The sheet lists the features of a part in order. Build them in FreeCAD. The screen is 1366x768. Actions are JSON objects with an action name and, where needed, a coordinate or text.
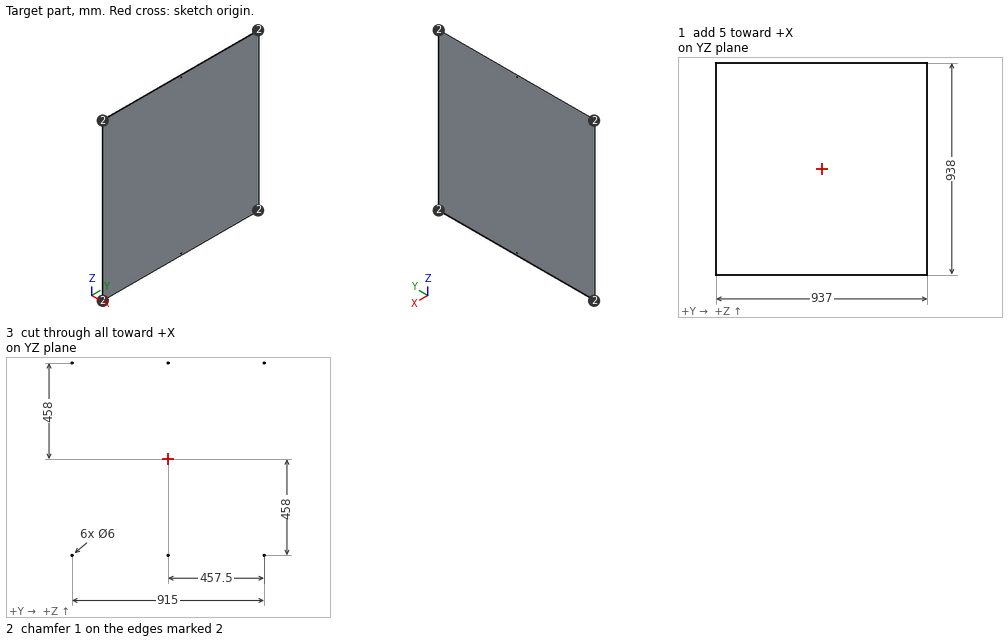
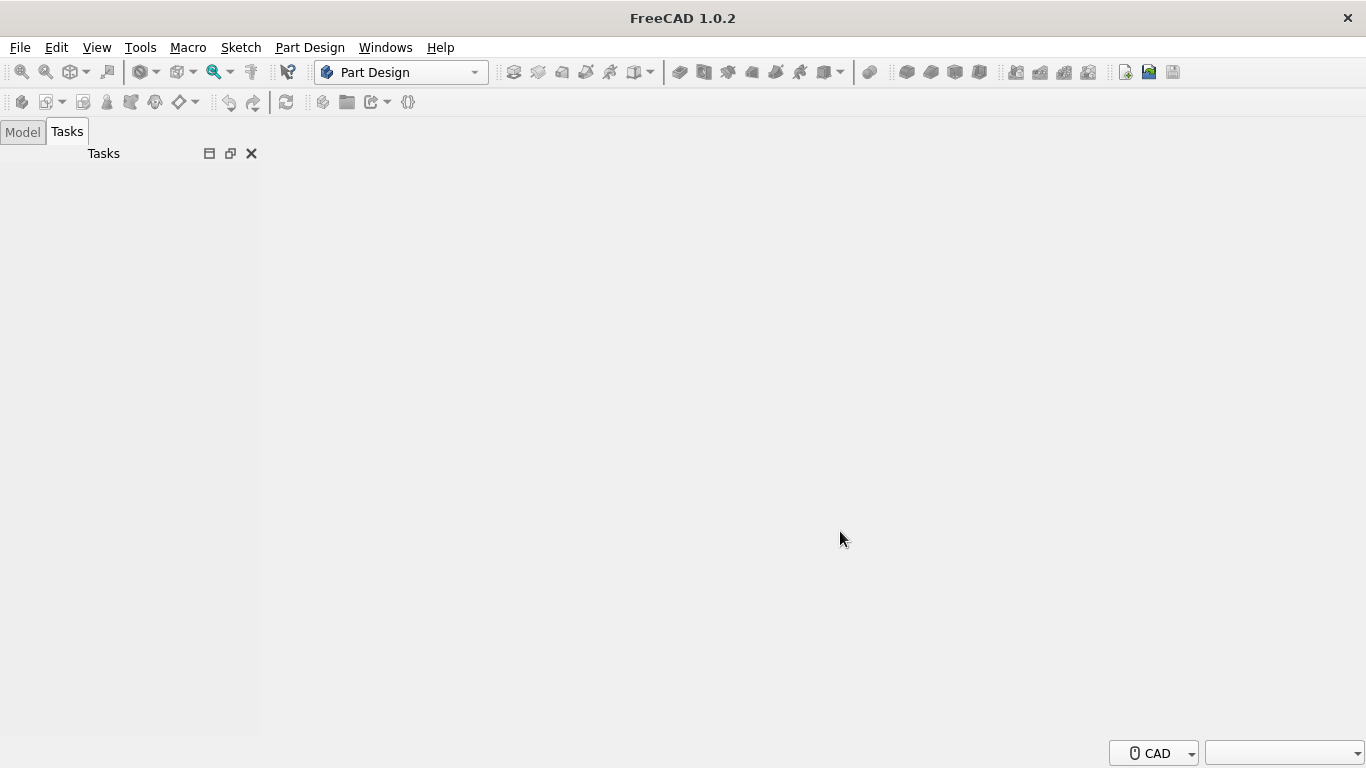
{"action": "left_click", "coordinate": [1126, 72]}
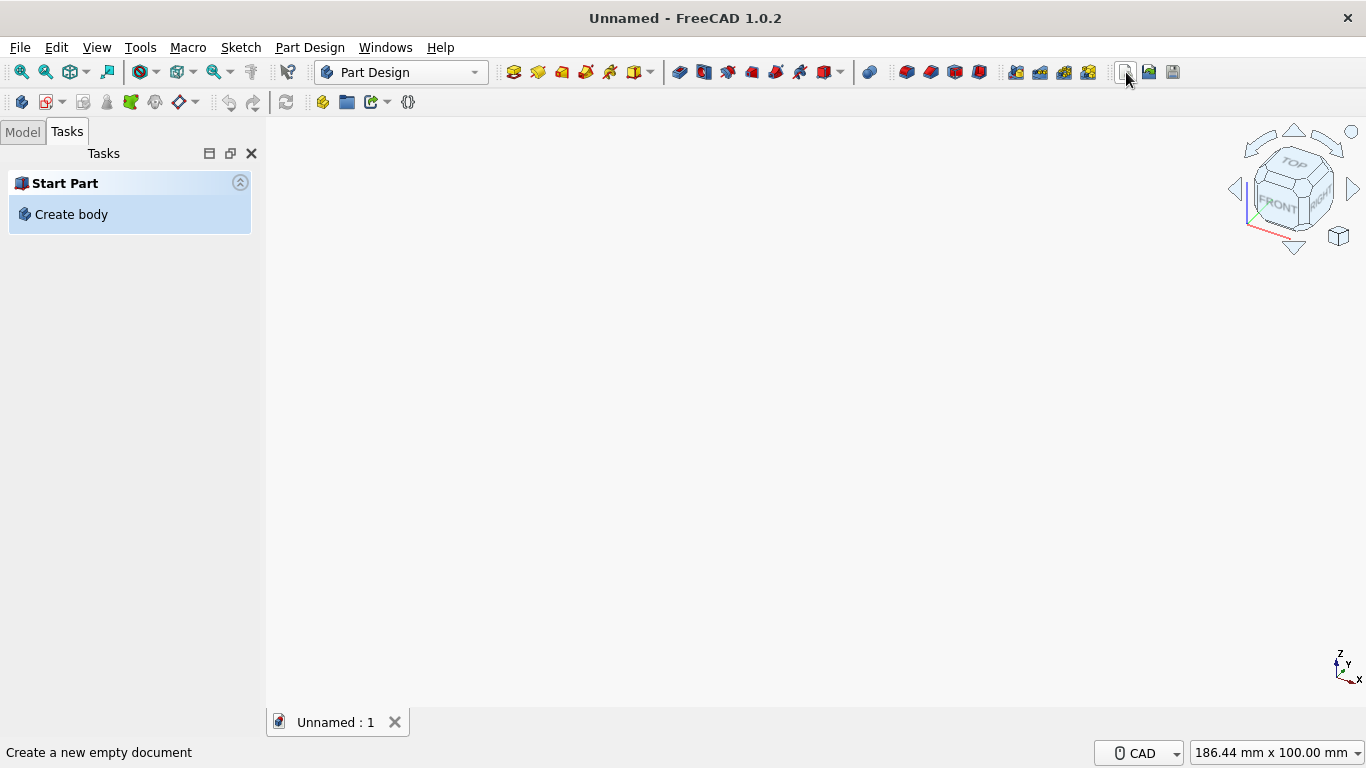
{"action": "left_click", "coordinate": [46, 102]}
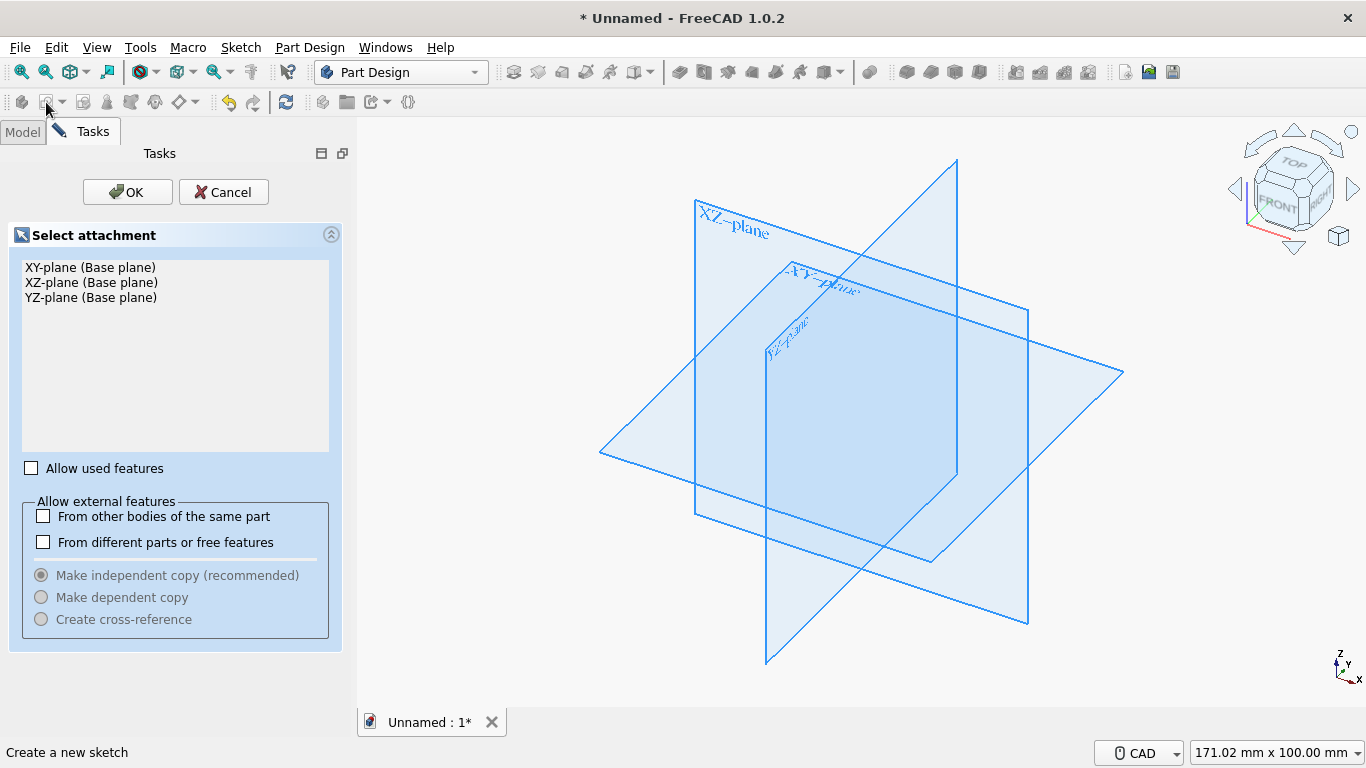
{"action": "left_click", "coordinate": [82, 298]}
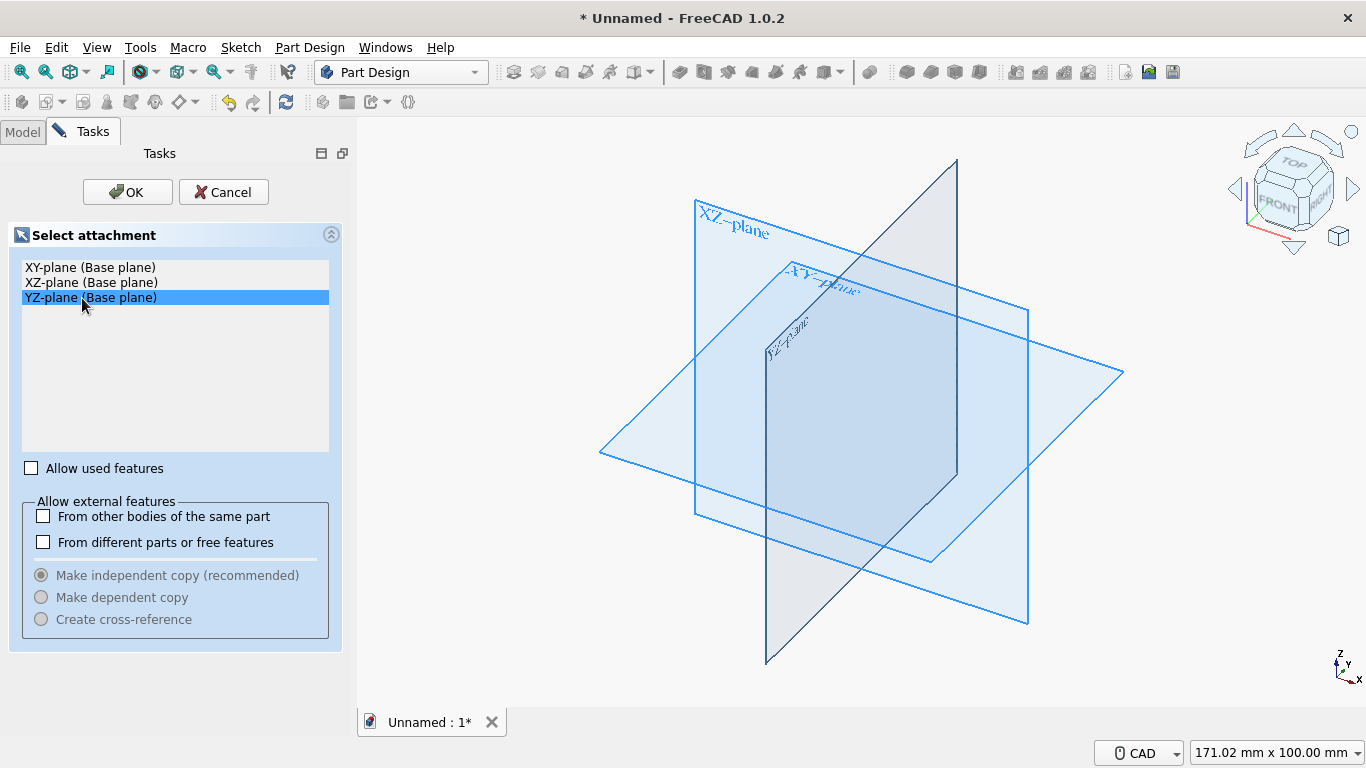
{"action": "left_click", "coordinate": [128, 192]}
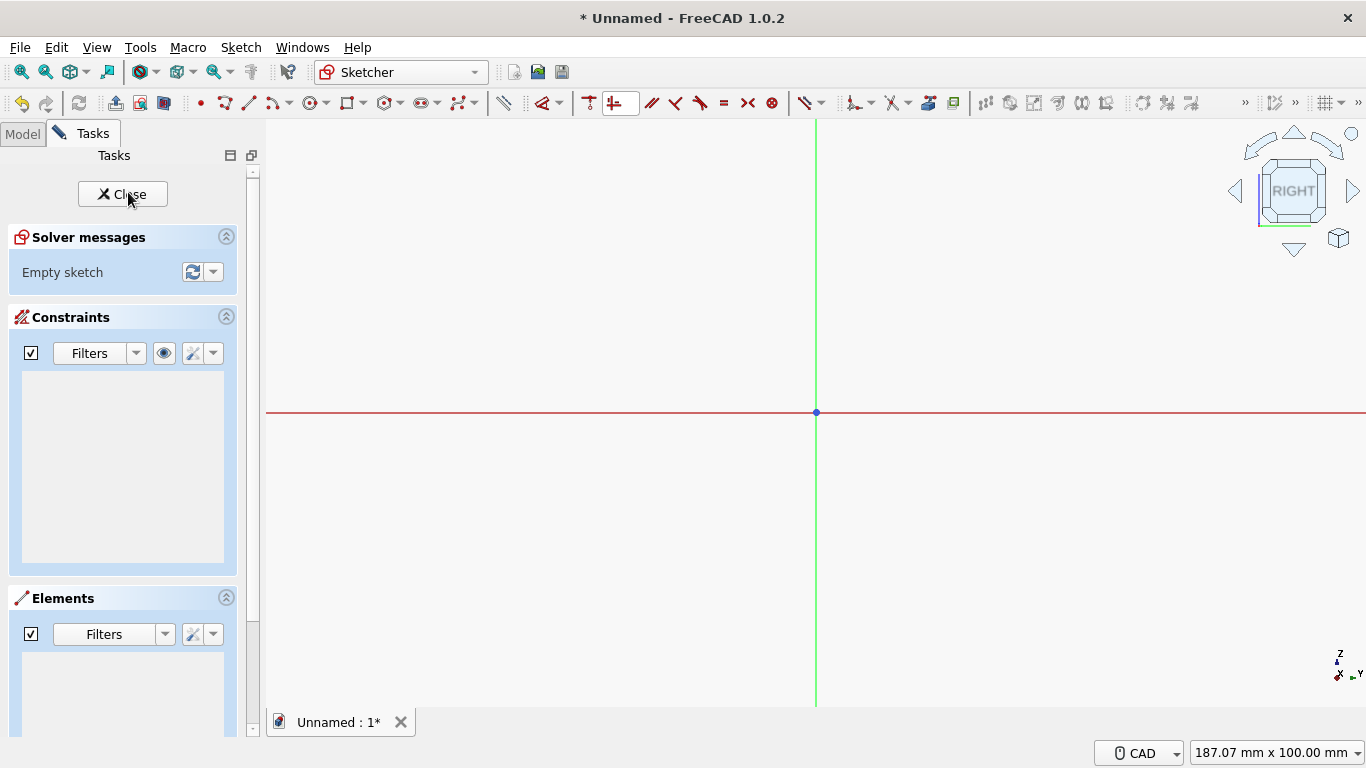
{"action": "scroll", "coordinate": [742, 413], "scroll_direction": "down", "scroll_amount": 13}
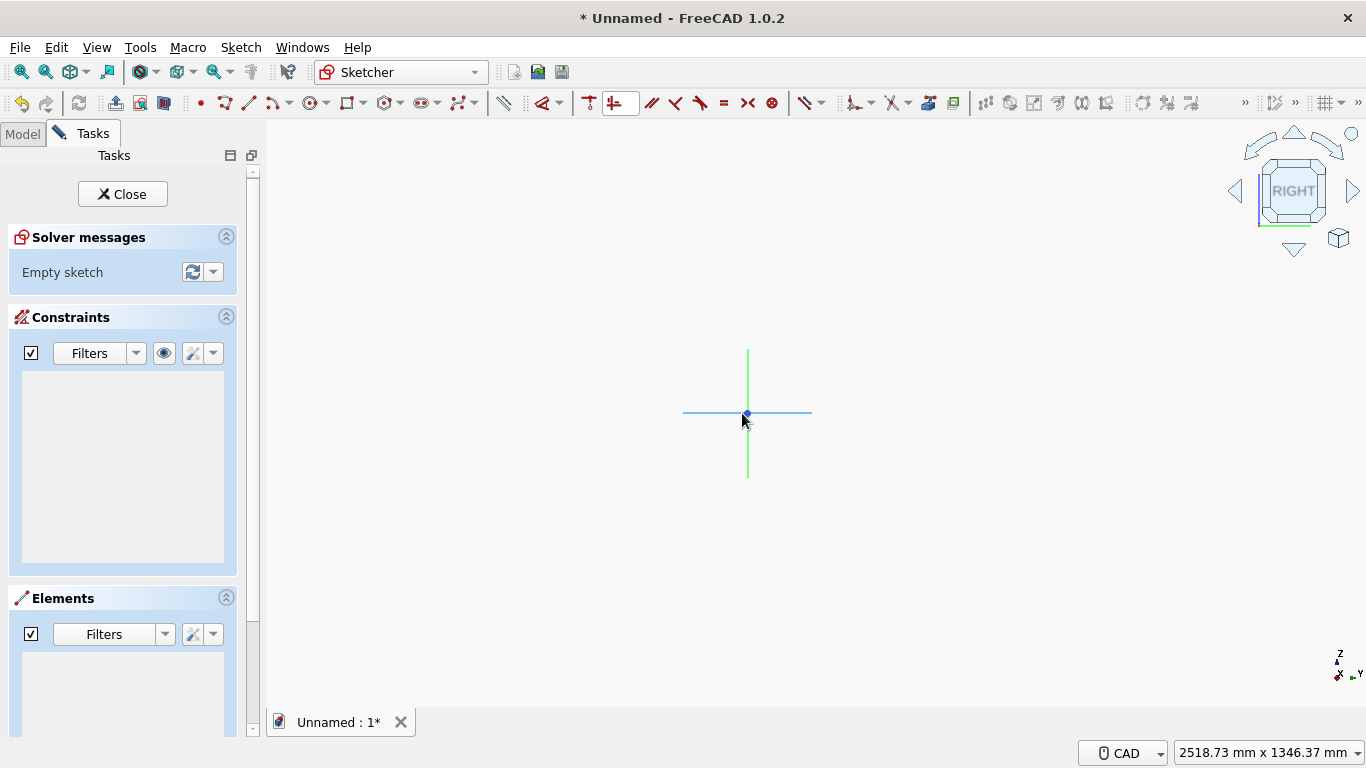
{"action": "left_click", "coordinate": [366, 104]}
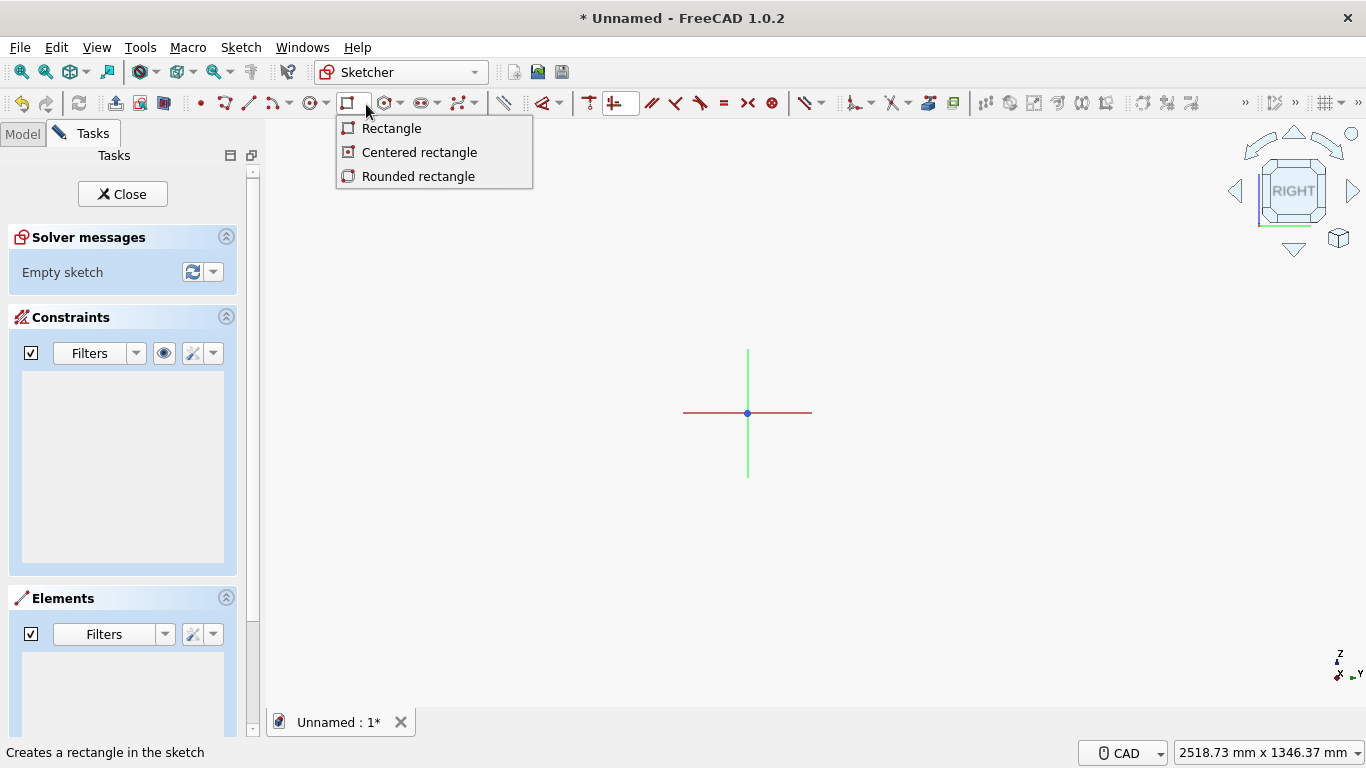
{"action": "left_click", "coordinate": [434, 152]}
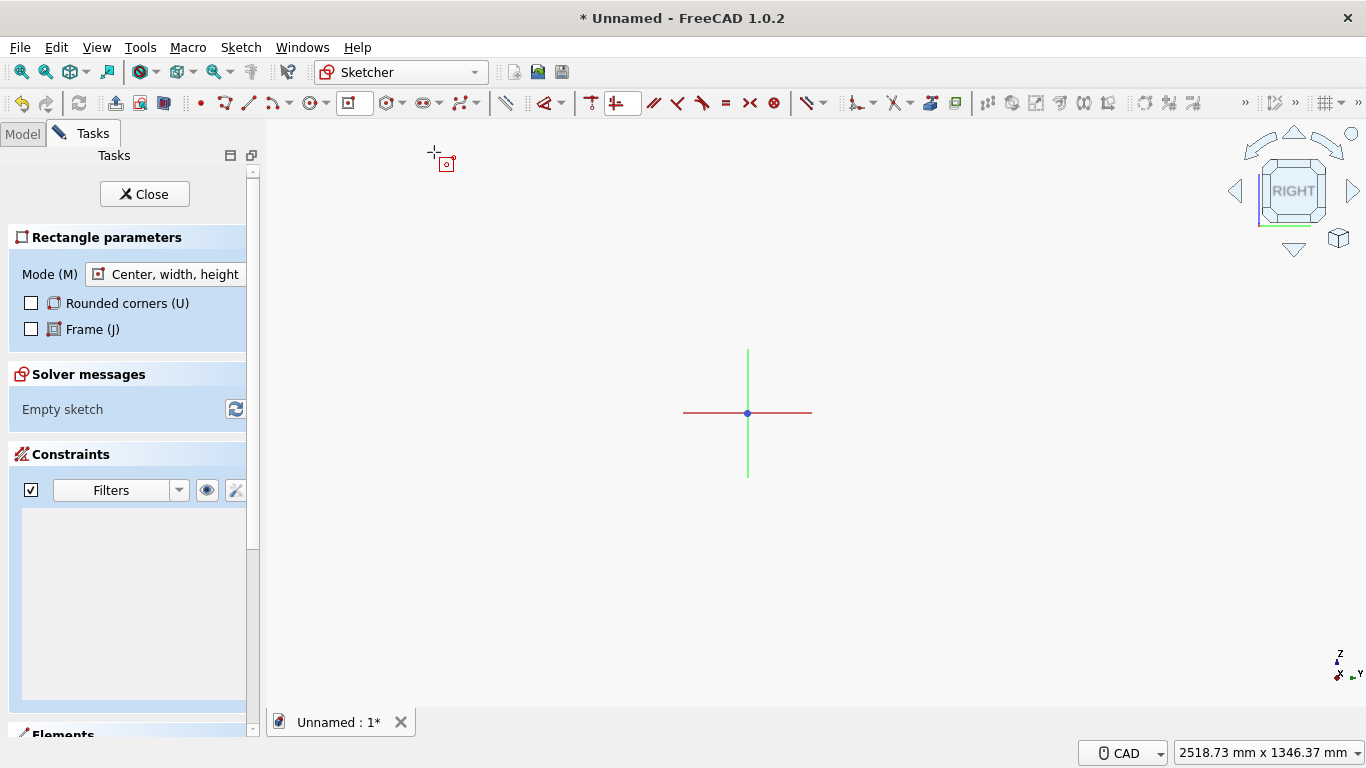
{"action": "left_click", "coordinate": [748, 413]}
{"action": "mouse_move", "coordinate": [953, 209]}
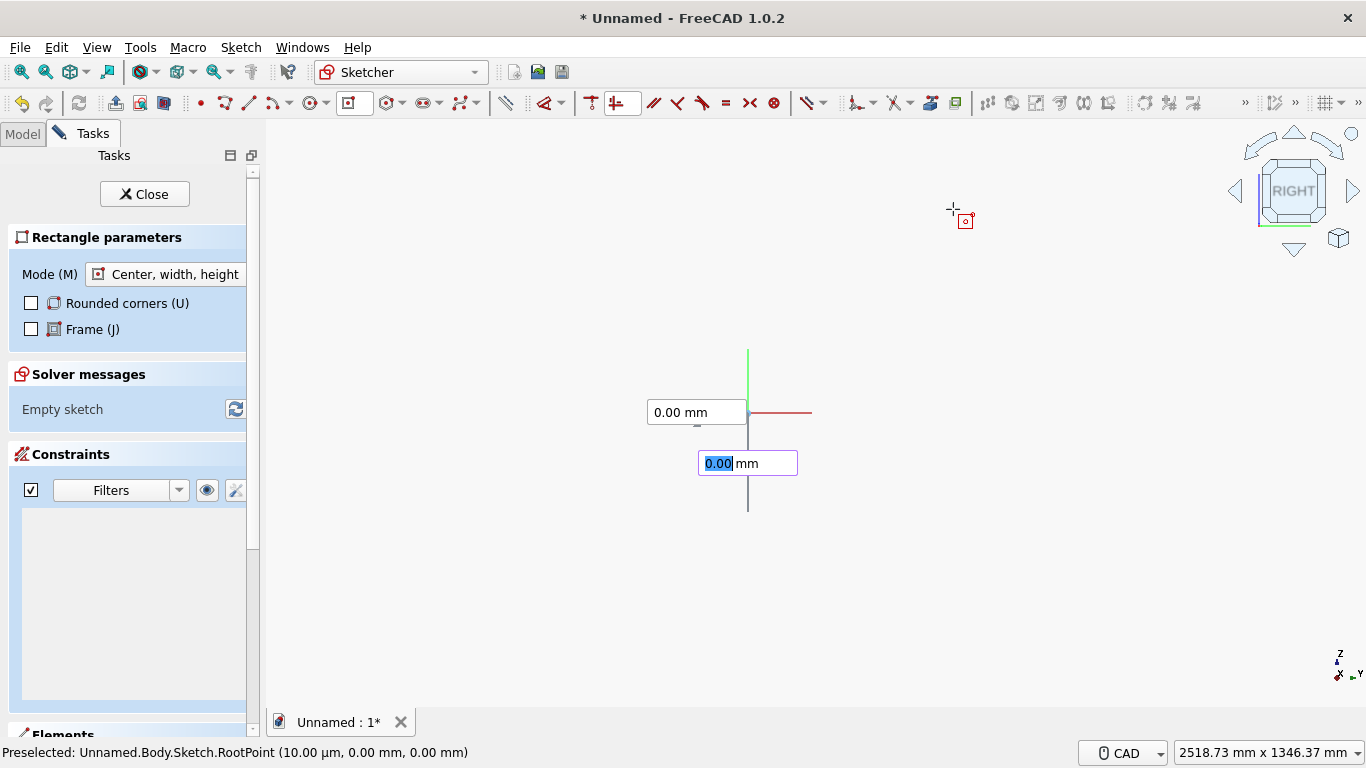
{"action": "type", "text": "937"}
{"action": "key", "text": "Tab"}
{"action": "type", "text": "938"}
{"action": "key", "text": "Return"}
{"action": "key", "text": "Escape"}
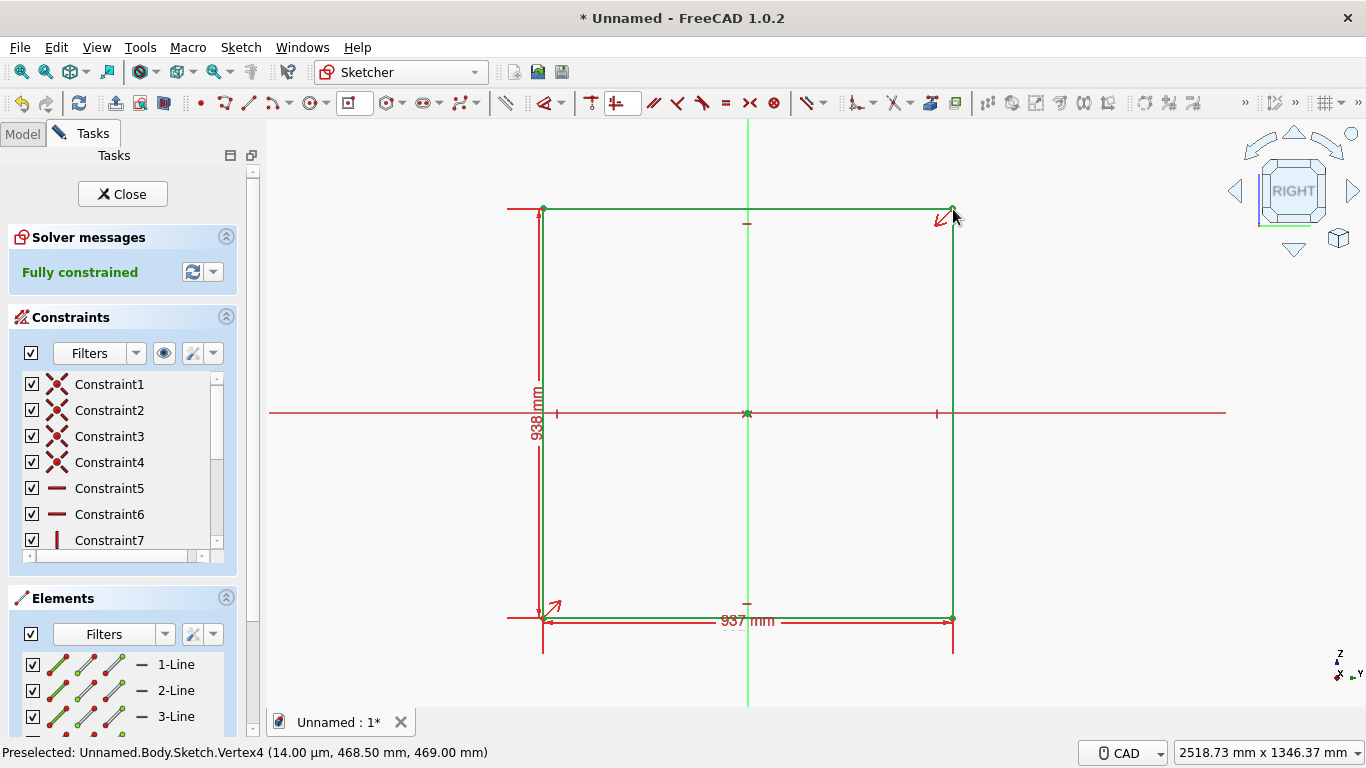
{"action": "left_click", "coordinate": [123, 194]}